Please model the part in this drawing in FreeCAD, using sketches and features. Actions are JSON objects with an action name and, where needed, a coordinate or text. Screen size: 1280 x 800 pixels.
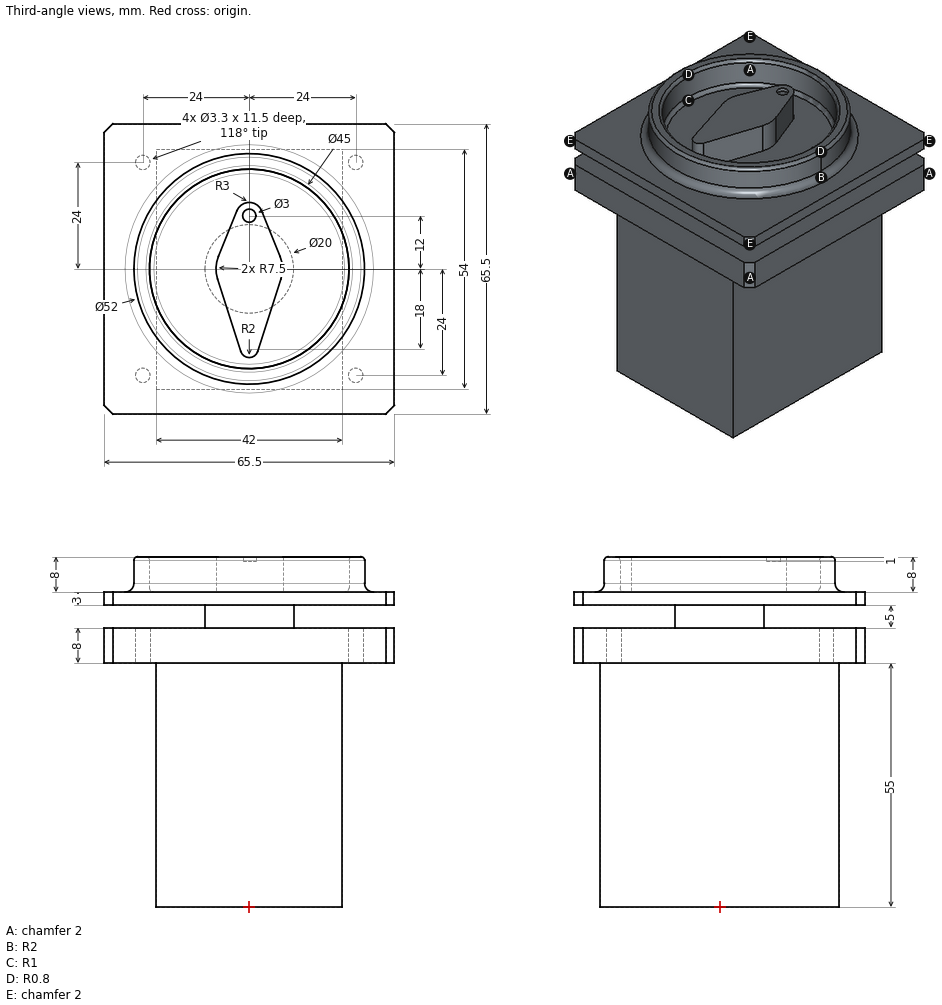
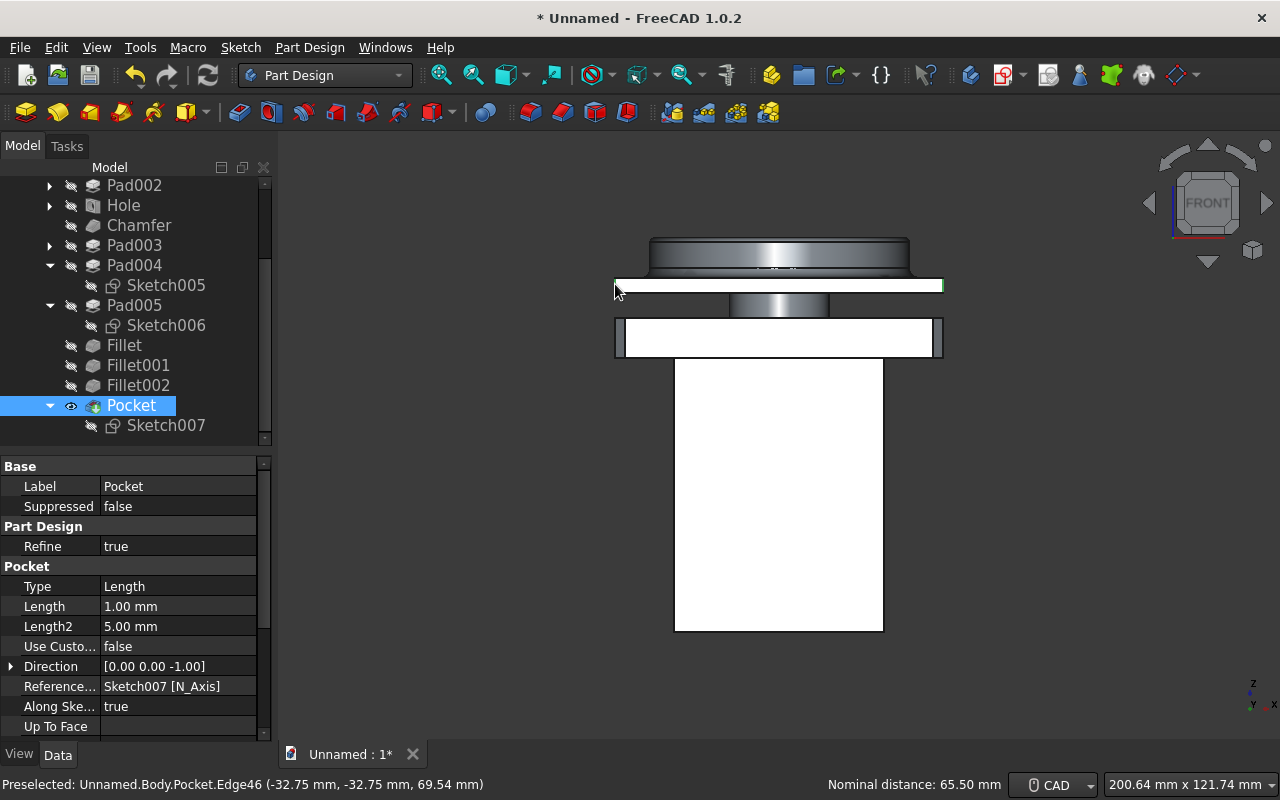
{"action": "scroll", "coordinate": [943, 284], "scroll_direction": "up", "scroll_amount": 5}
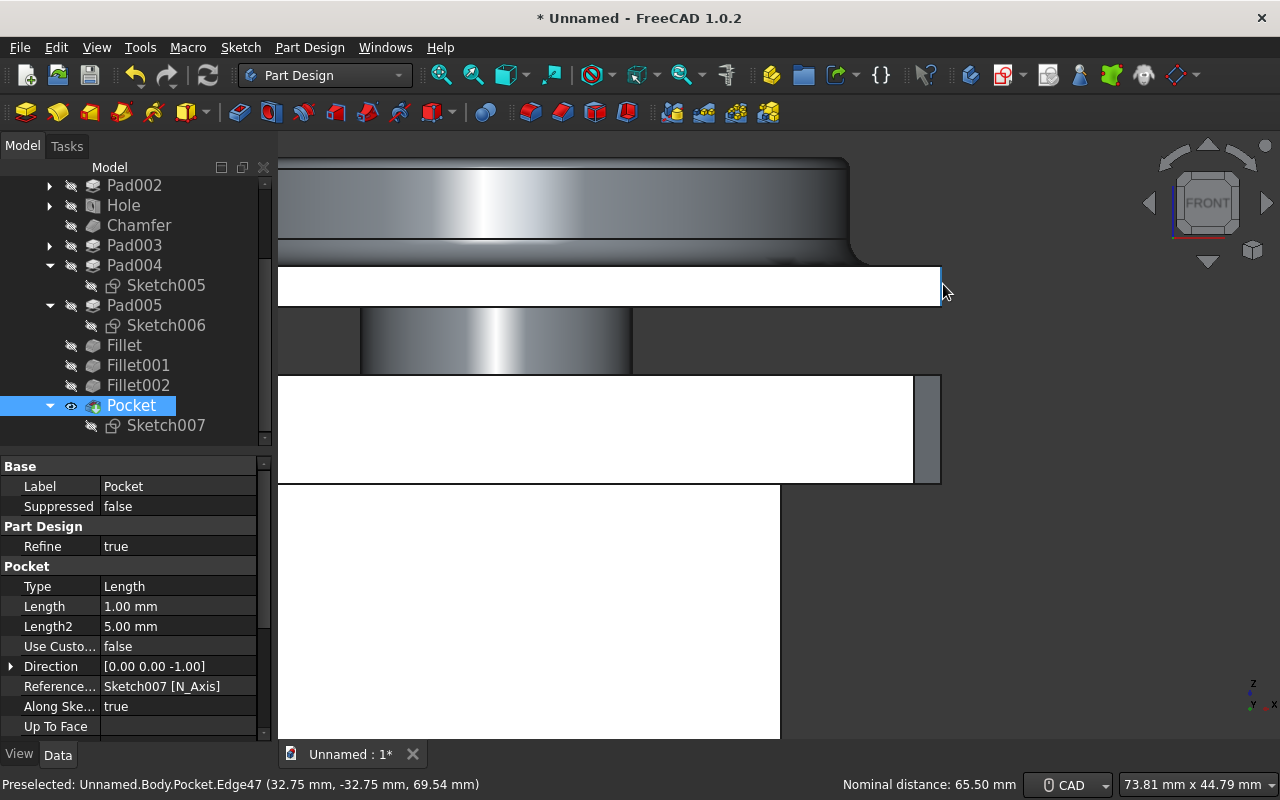
{"action": "left_click", "coordinate": [442, 76]}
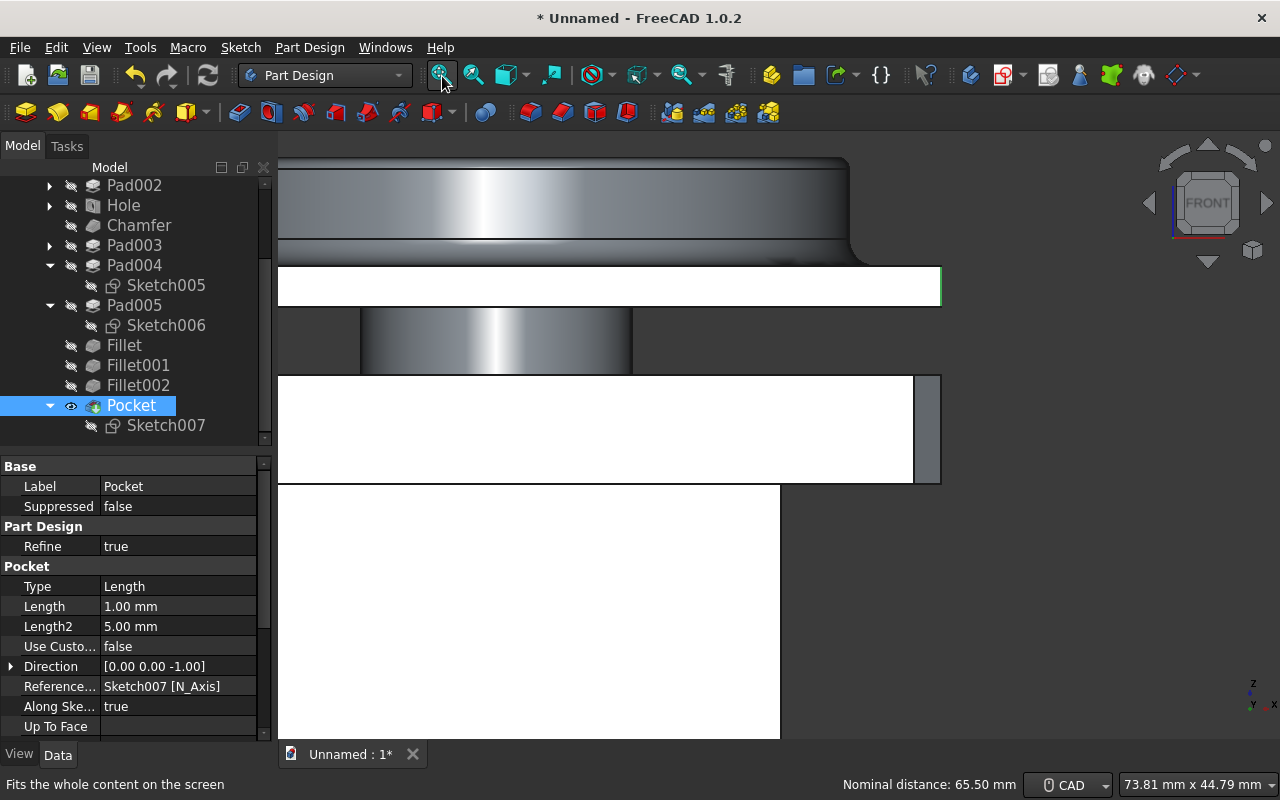
{"action": "key", "text": "3"}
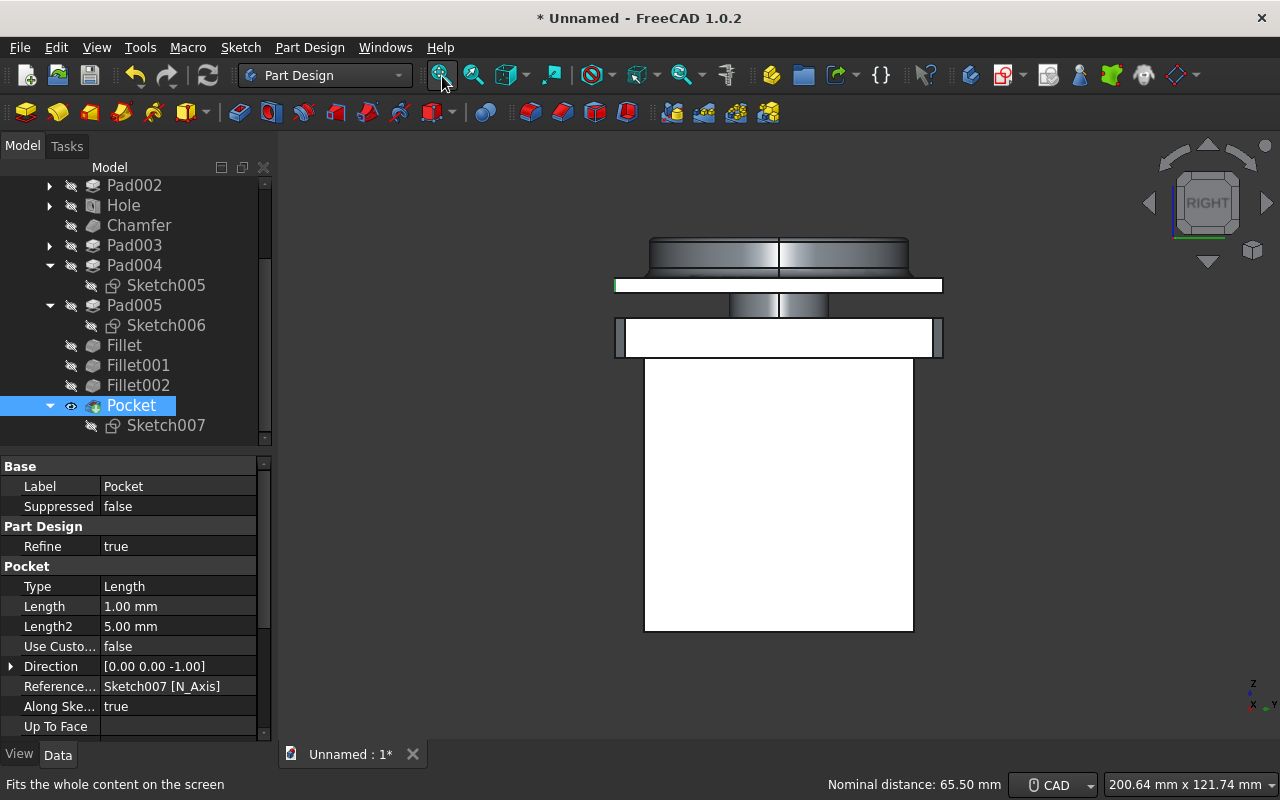
{"action": "left_click", "coordinate": [943, 284], "text": "ctrl"}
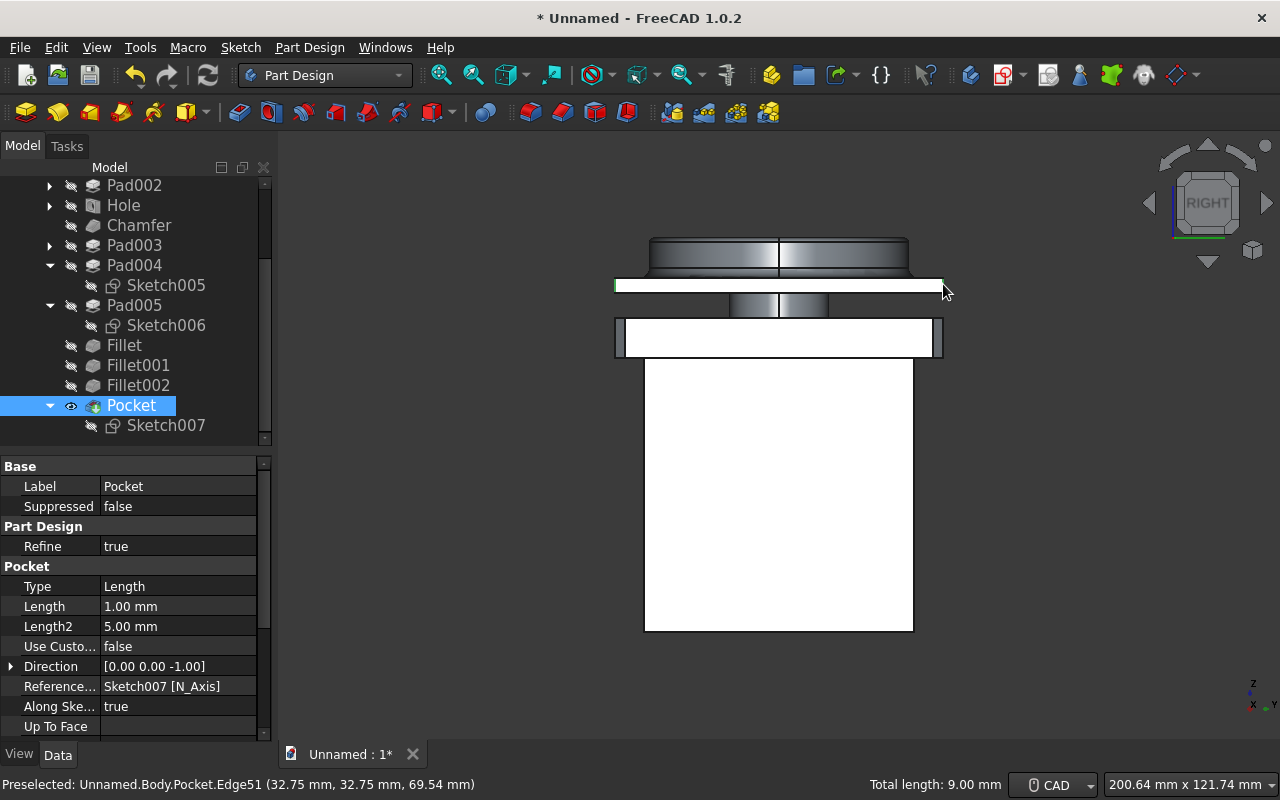
{"action": "scroll", "coordinate": [943, 284], "scroll_direction": "up", "scroll_amount": 5}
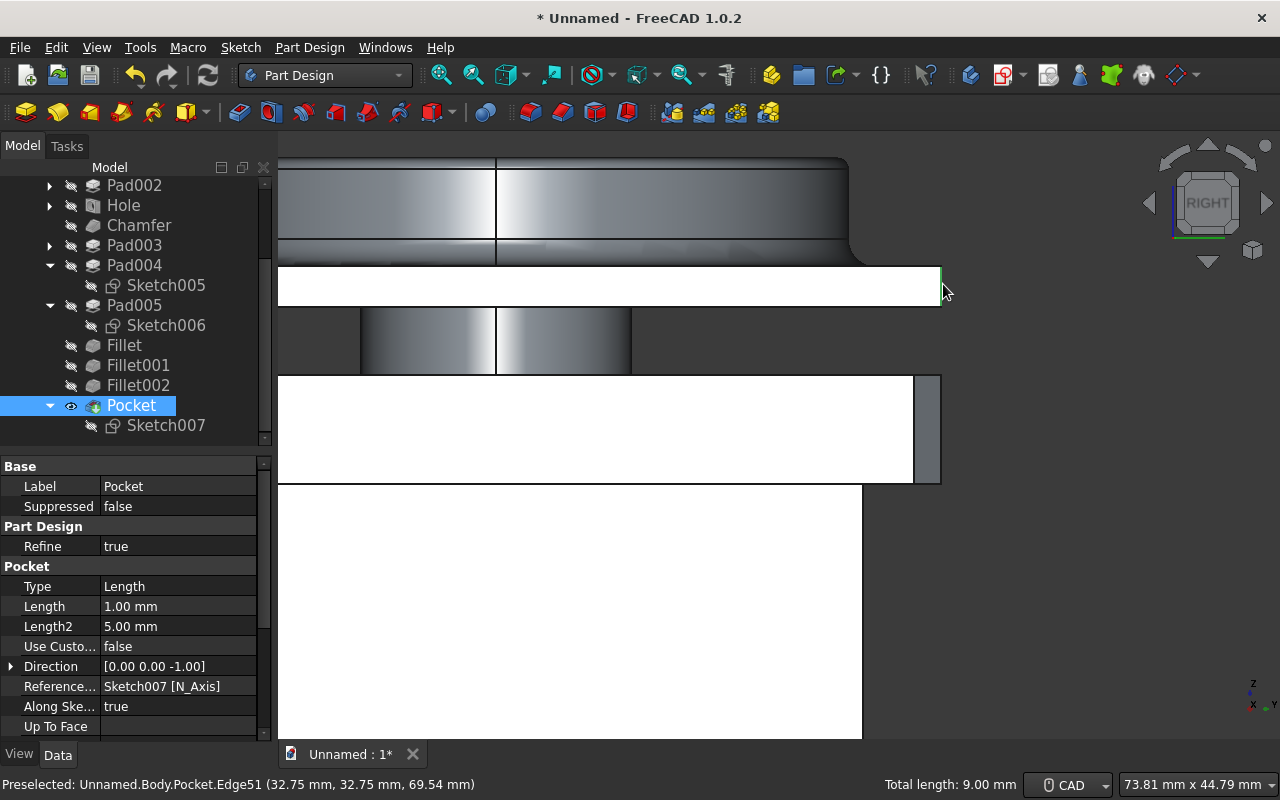
{"action": "left_click", "coordinate": [442, 76]}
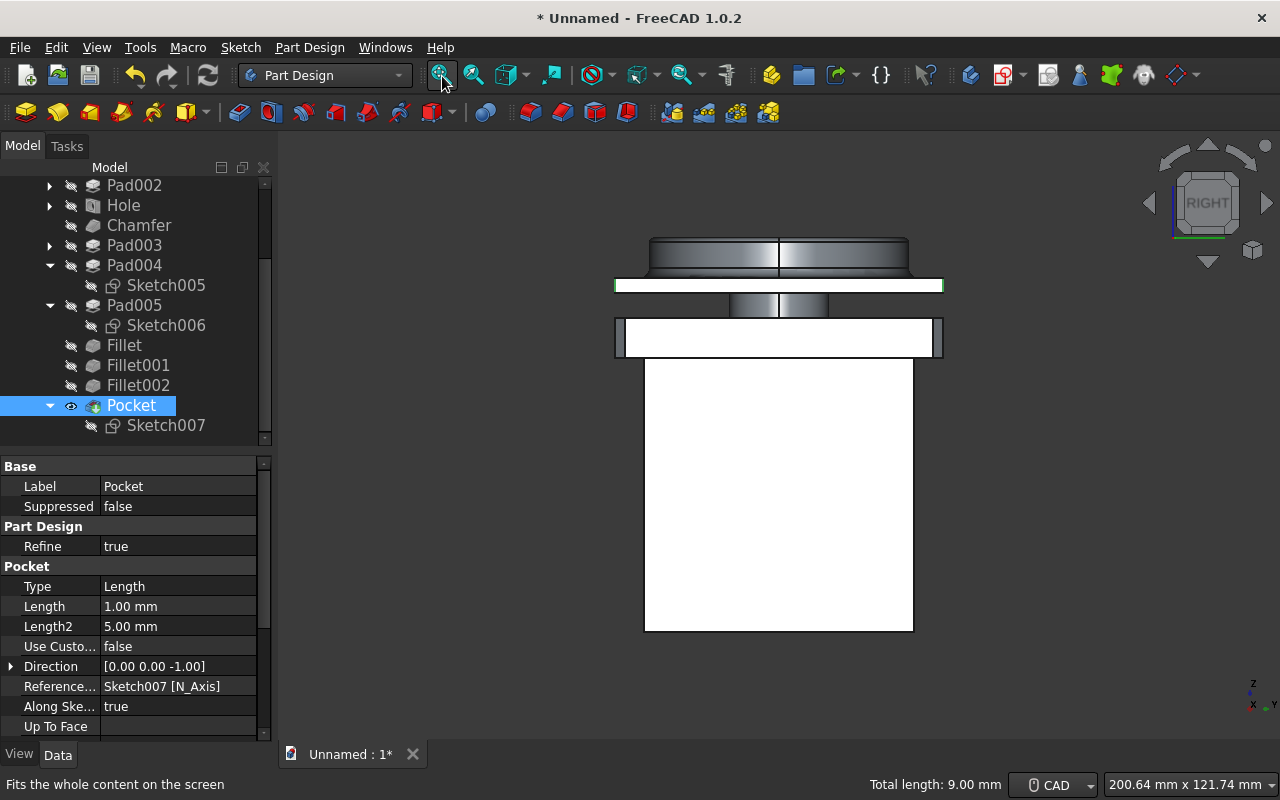
{"action": "key", "text": "5"}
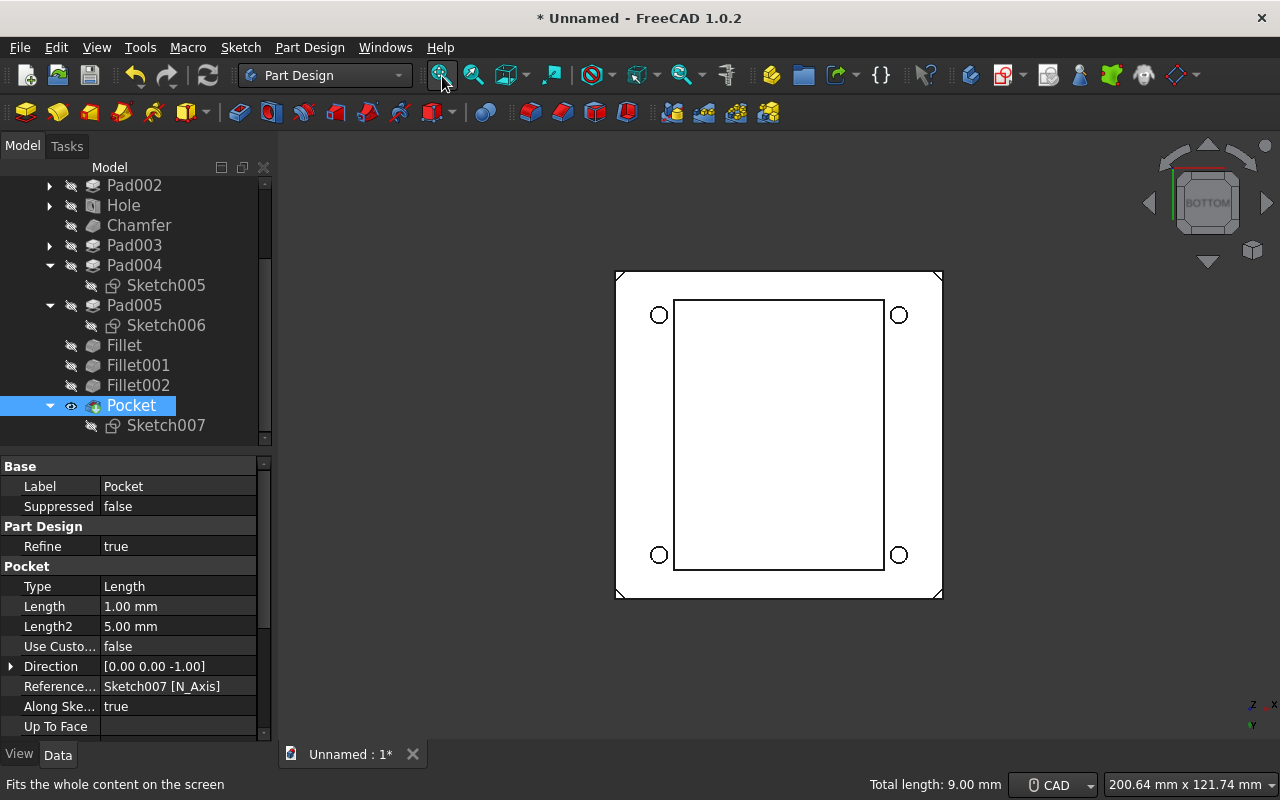
{"action": "scroll", "coordinate": [615, 598], "scroll_direction": "up", "scroll_amount": 5}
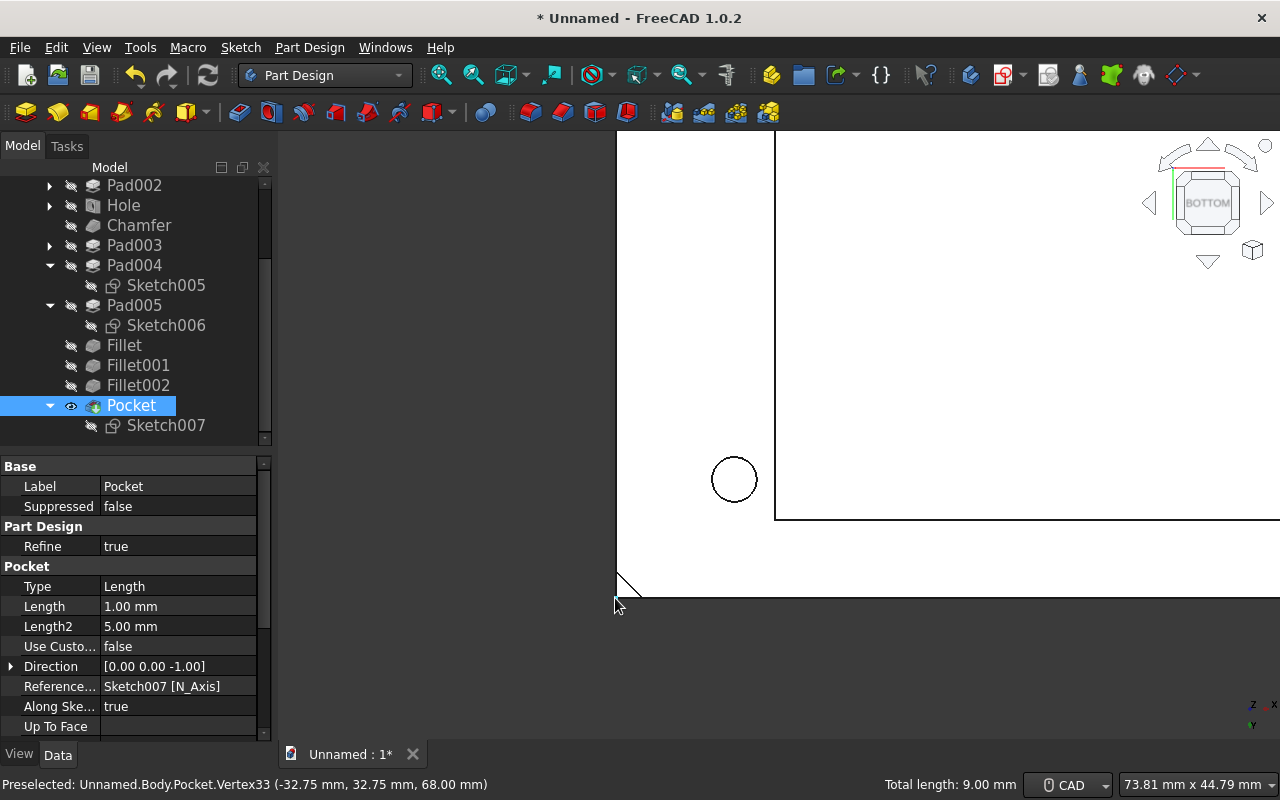
{"action": "left_click", "coordinate": [442, 76]}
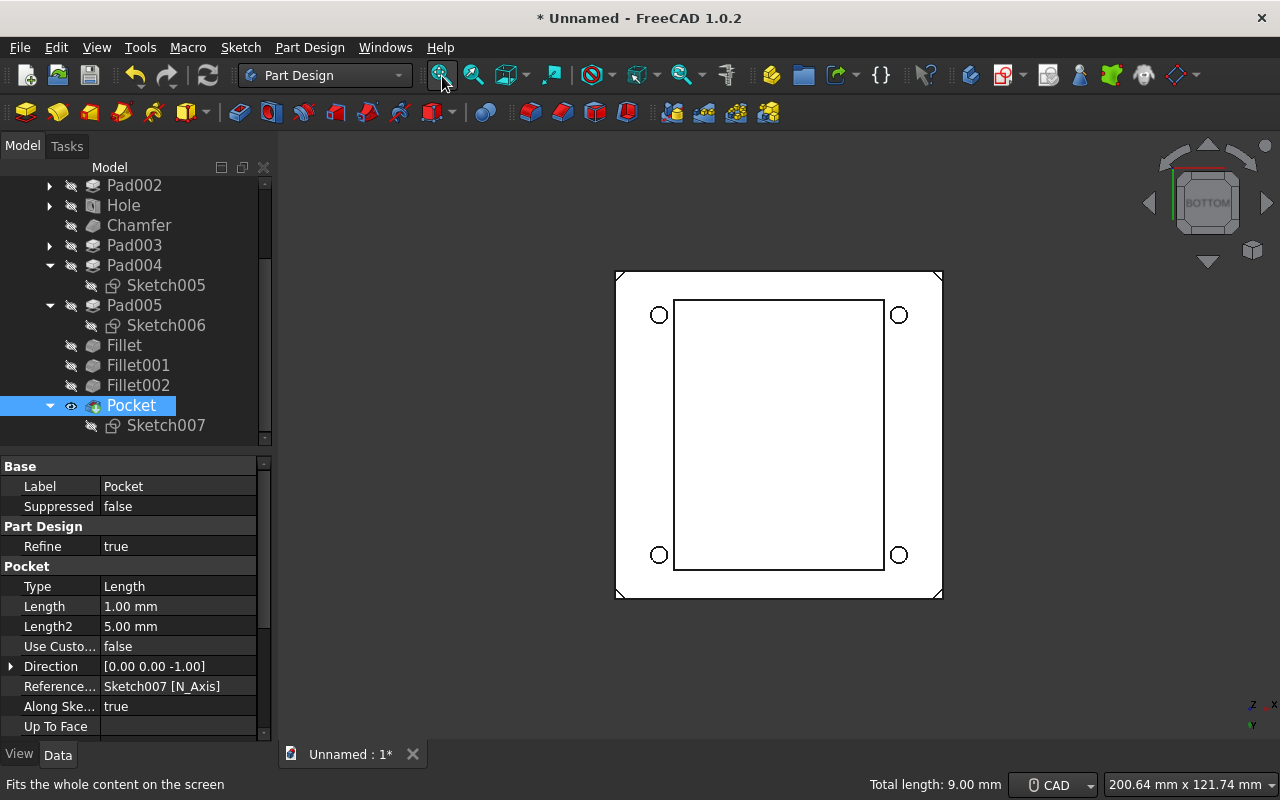
{"action": "key", "text": "4"}